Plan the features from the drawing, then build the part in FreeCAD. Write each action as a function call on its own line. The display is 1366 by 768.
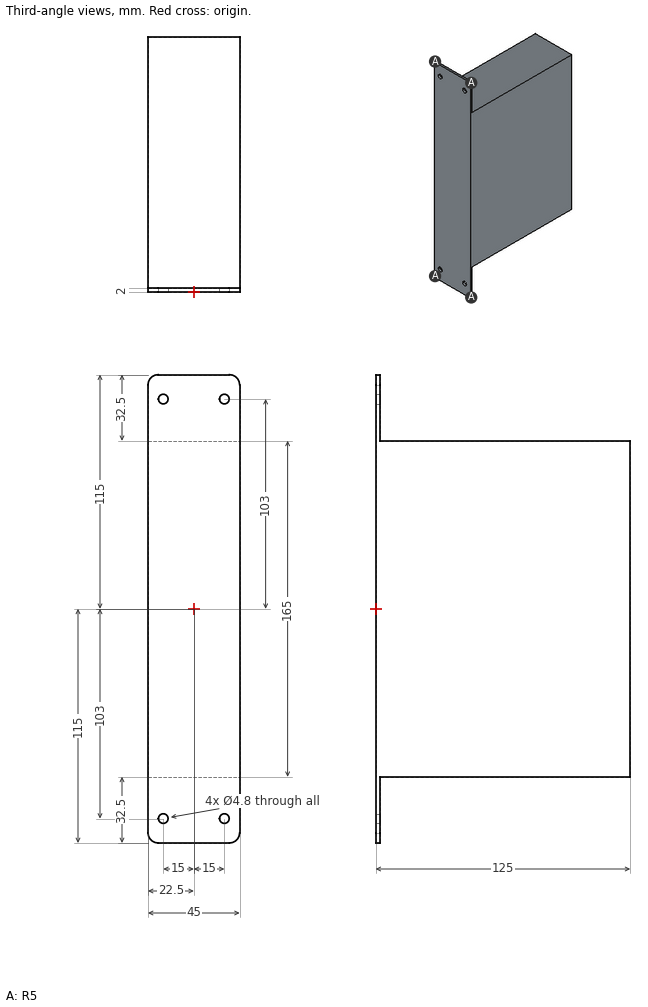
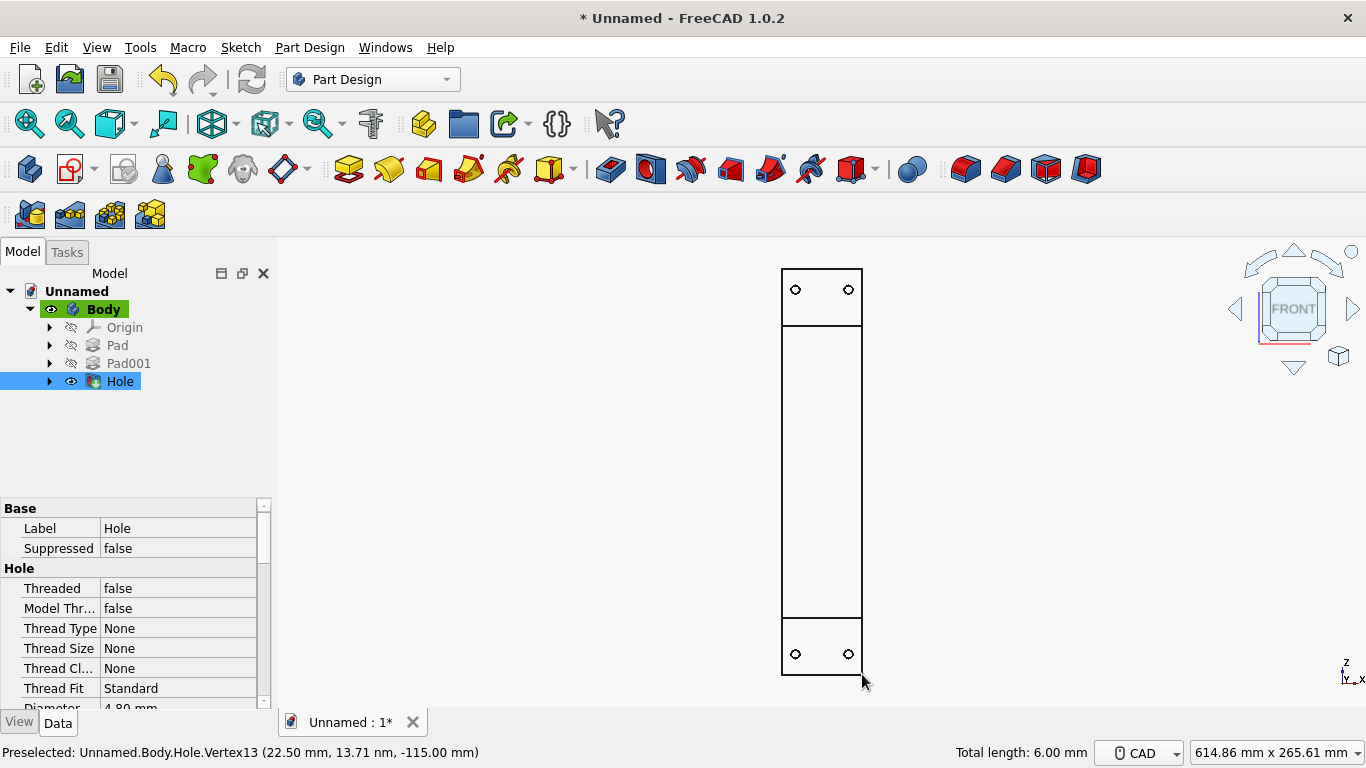
key(3)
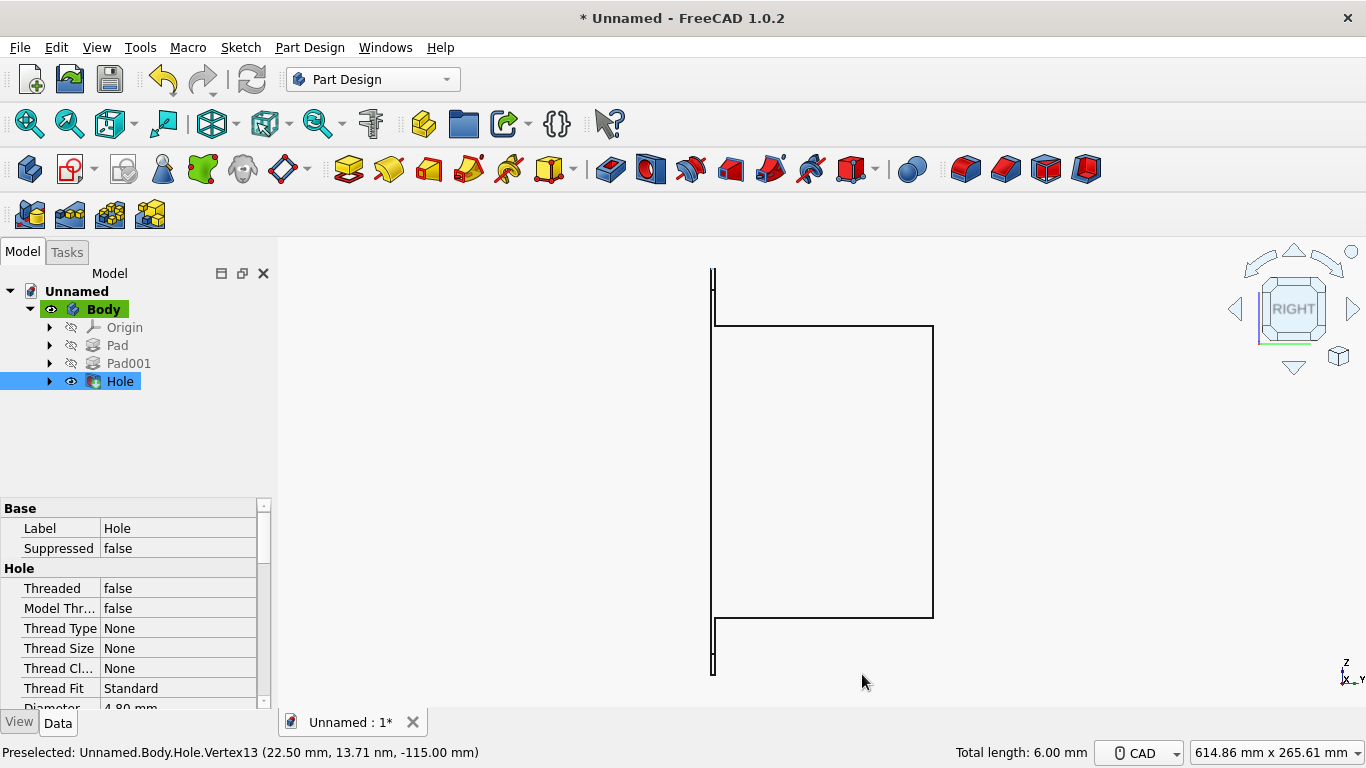
scroll(713, 674, up, 13)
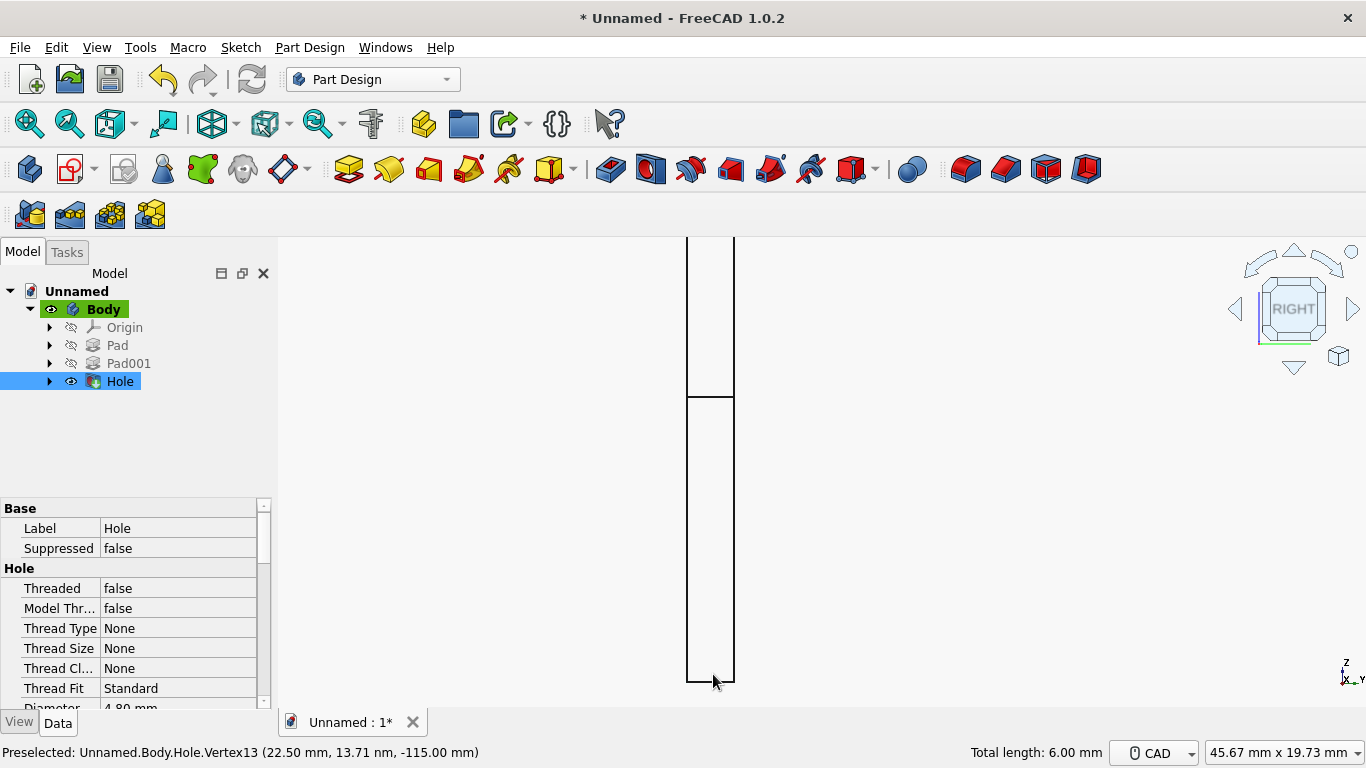
click(30, 124)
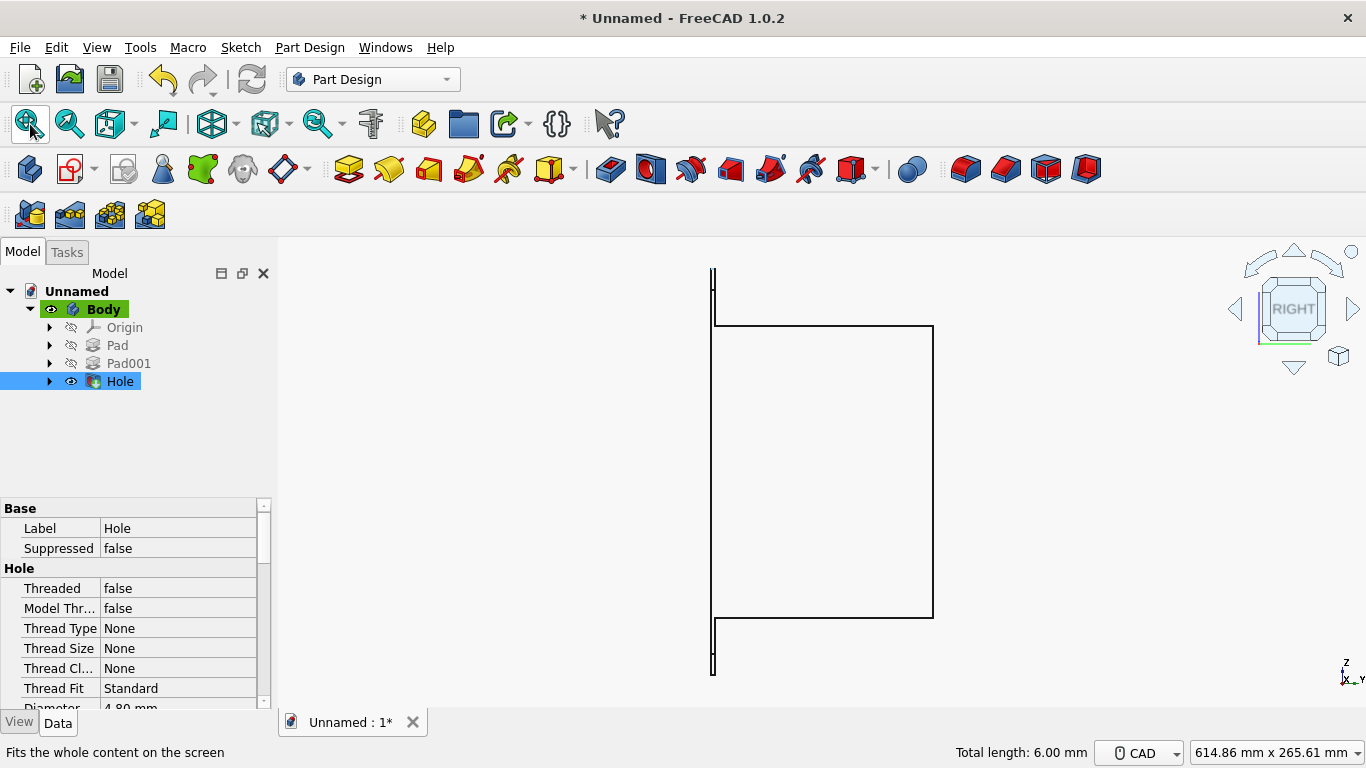
key(5)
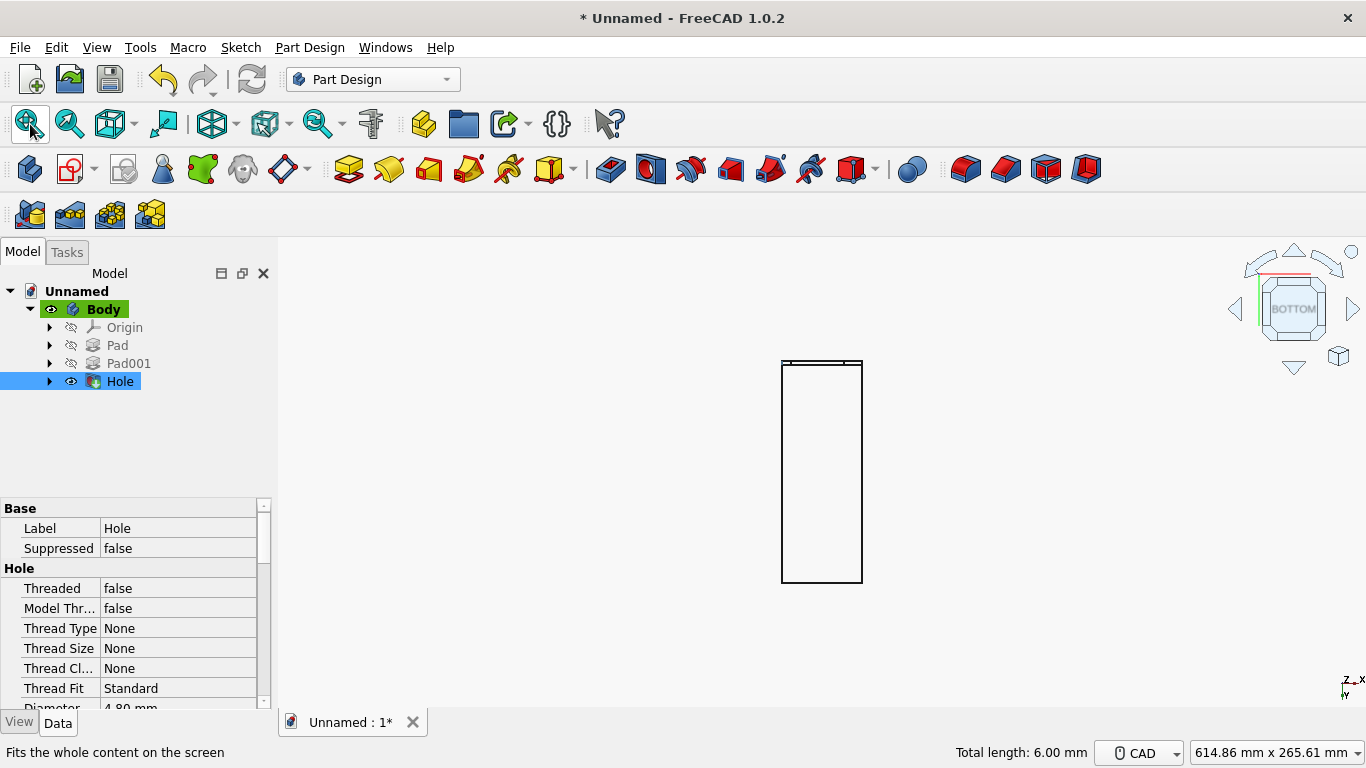
scroll(862, 362, up, 13)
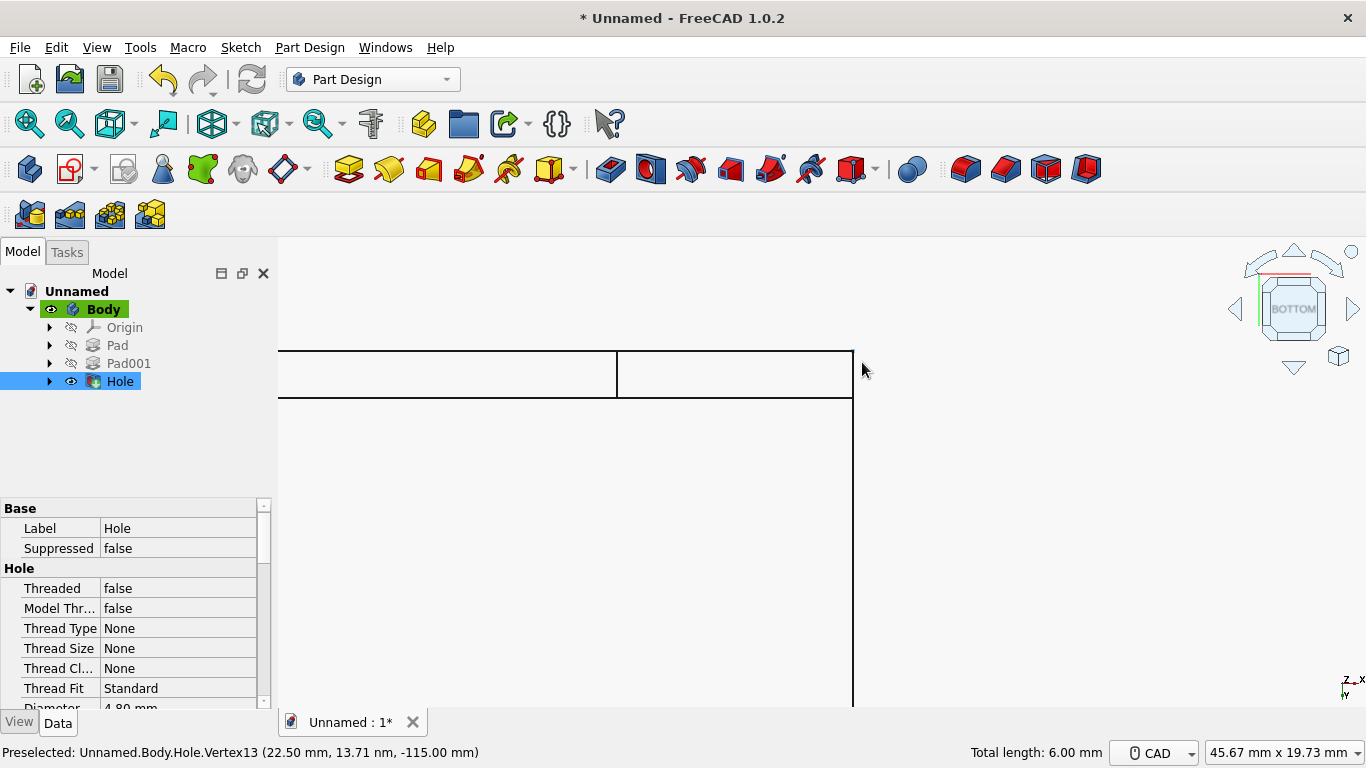
click(853, 374, ctrl)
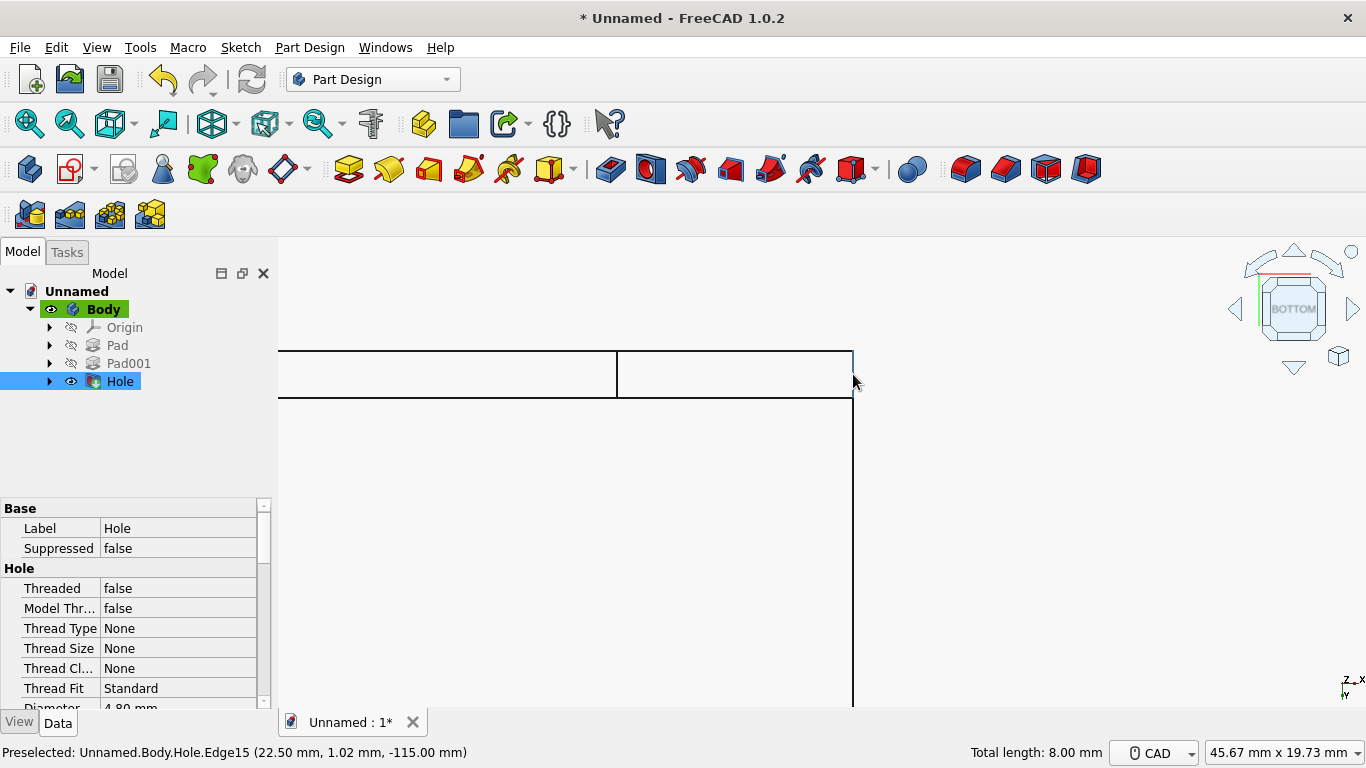
key(v)
key(1)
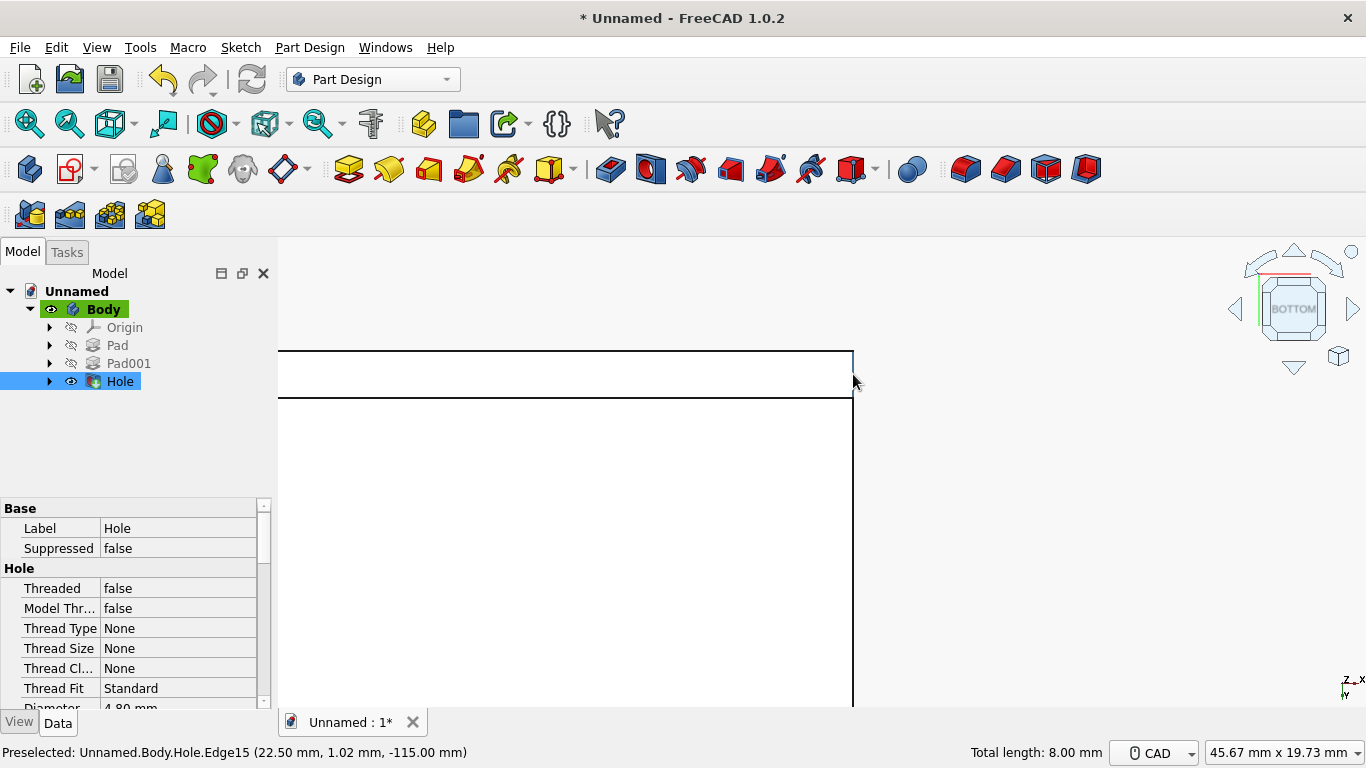
click(966, 170)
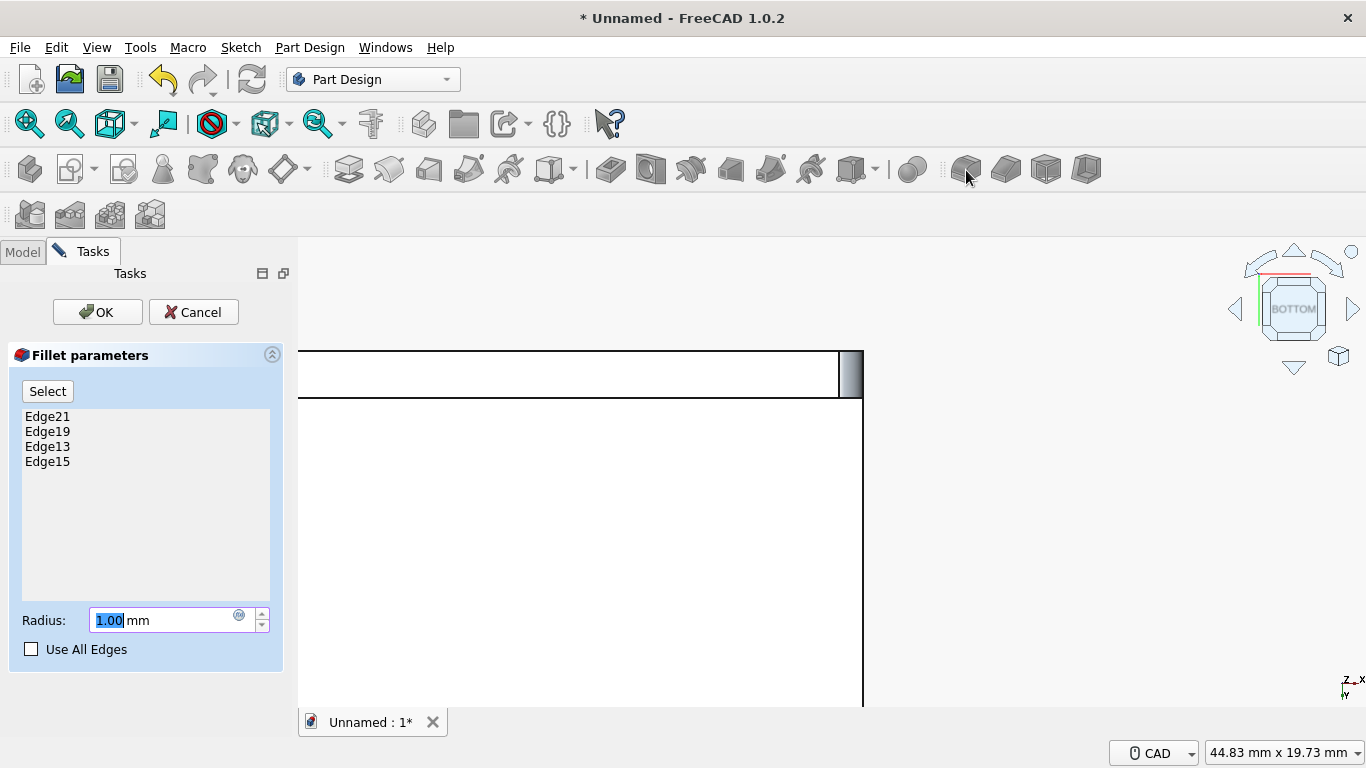
text(5)
key(Tab)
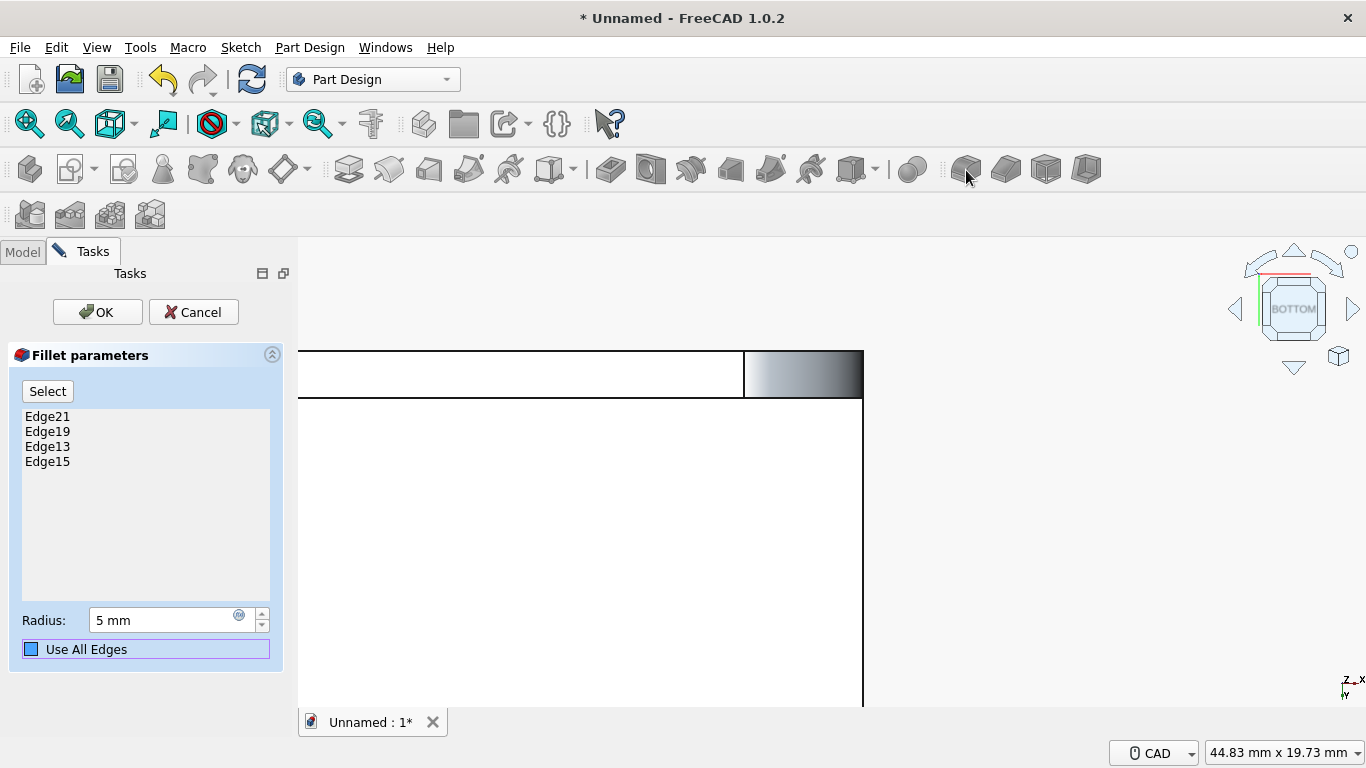
click(98, 312)